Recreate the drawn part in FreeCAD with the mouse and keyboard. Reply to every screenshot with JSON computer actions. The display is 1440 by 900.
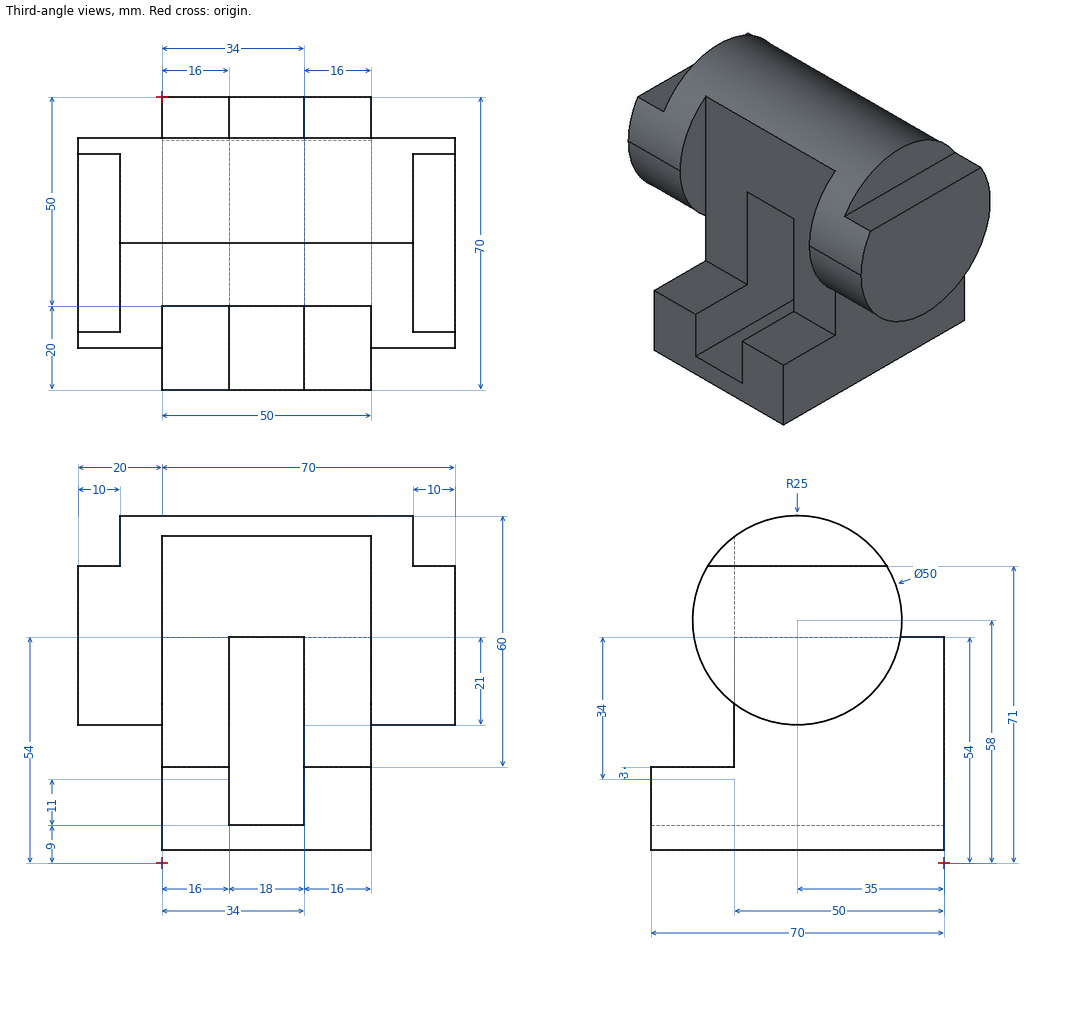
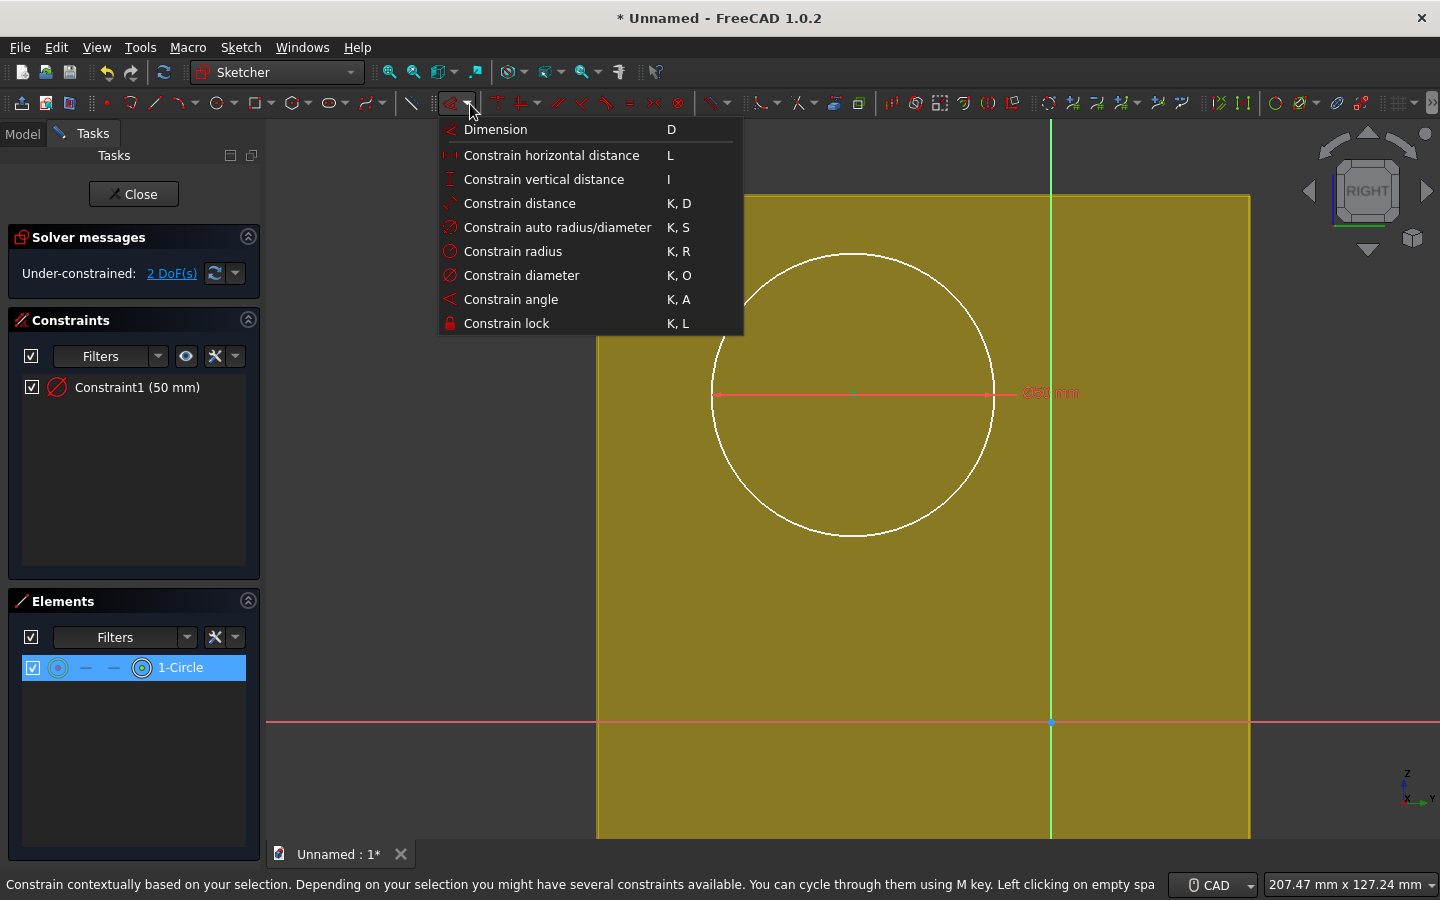
{"action": "left_click", "coordinate": [591, 155]}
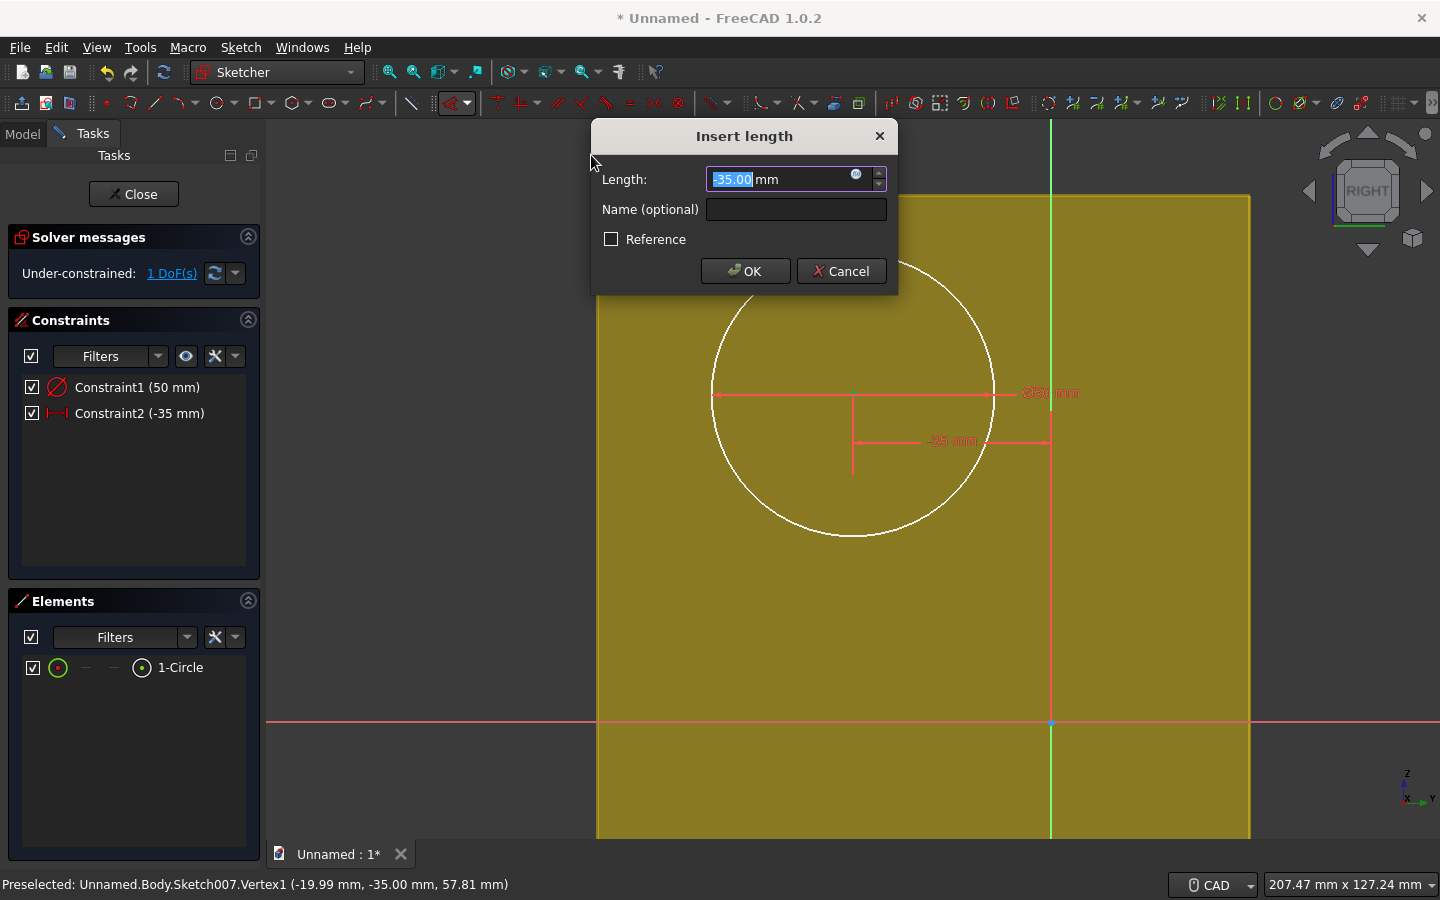
{"action": "type", "text": "-35"}
{"action": "key", "text": "Return"}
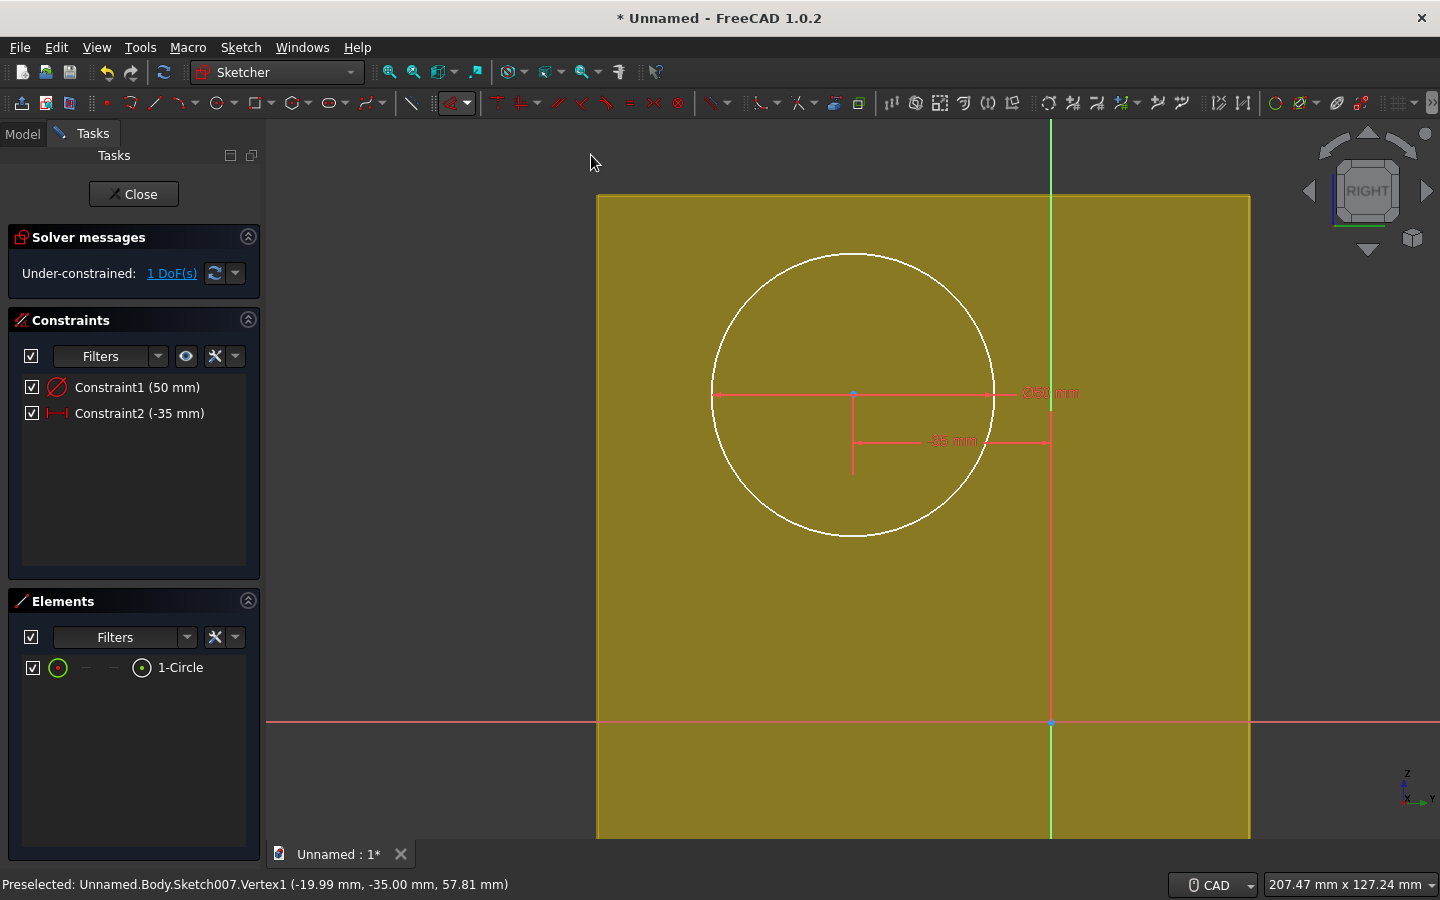
{"action": "left_click", "coordinate": [853, 395]}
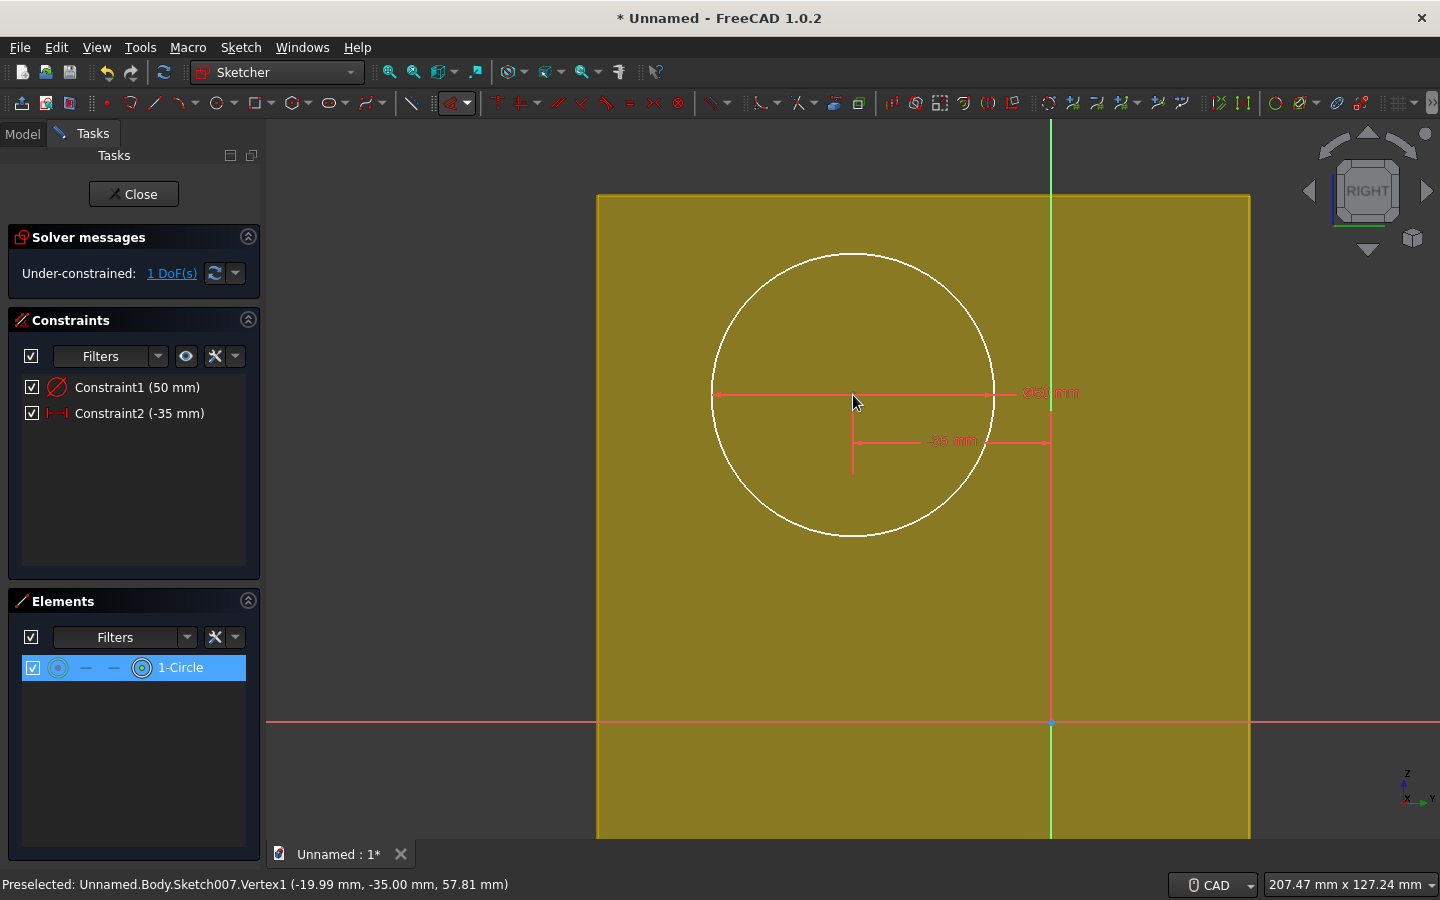
{"action": "left_click", "coordinate": [470, 104]}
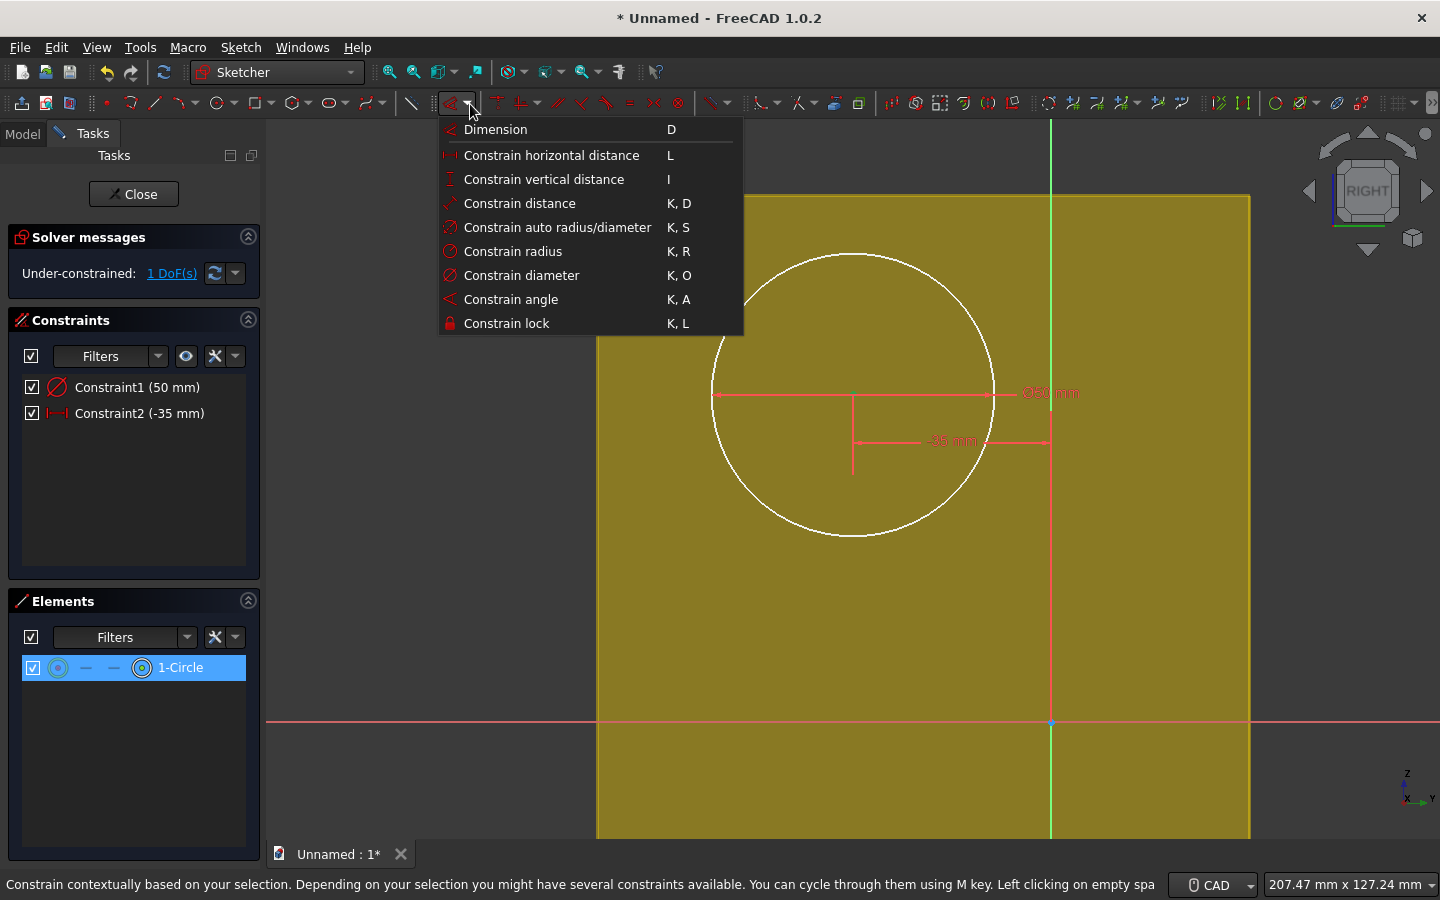
{"action": "left_click", "coordinate": [591, 179]}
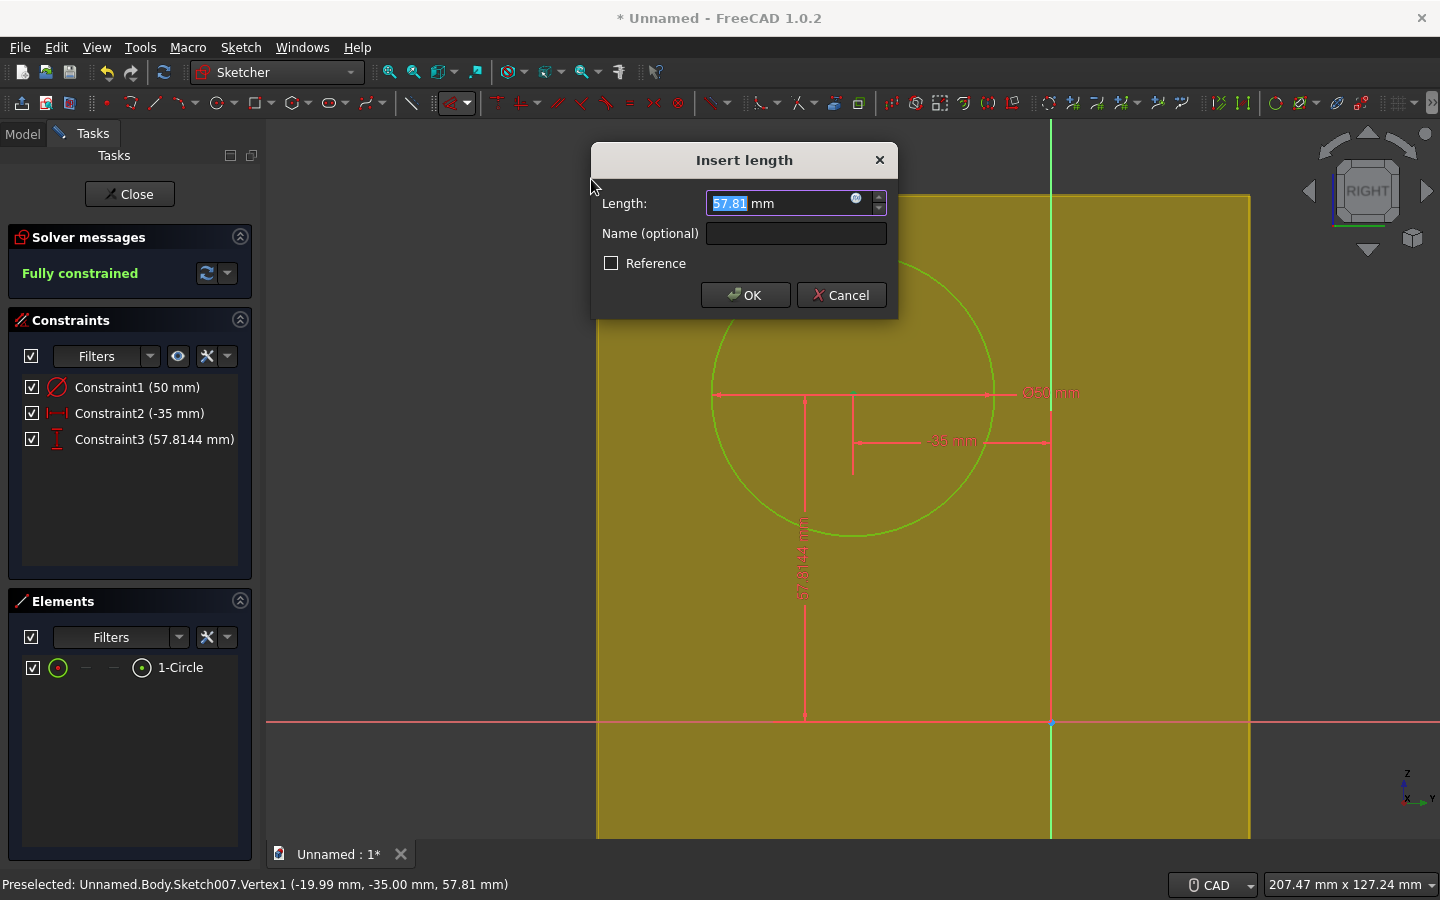
{"action": "type", "text": "58"}
{"action": "key", "text": "Return"}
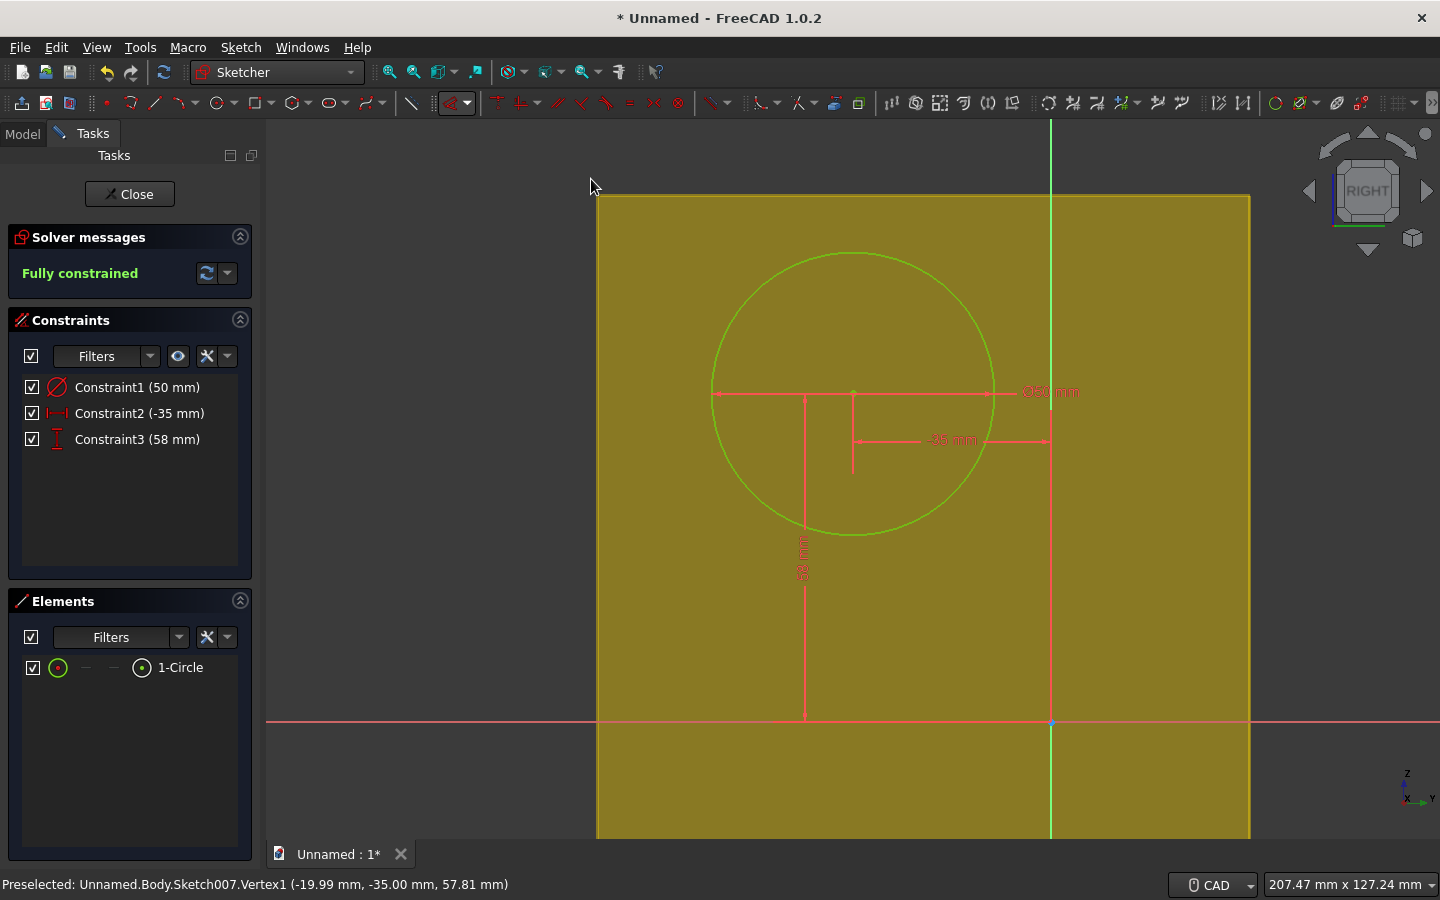
{"action": "left_click", "coordinate": [130, 194]}